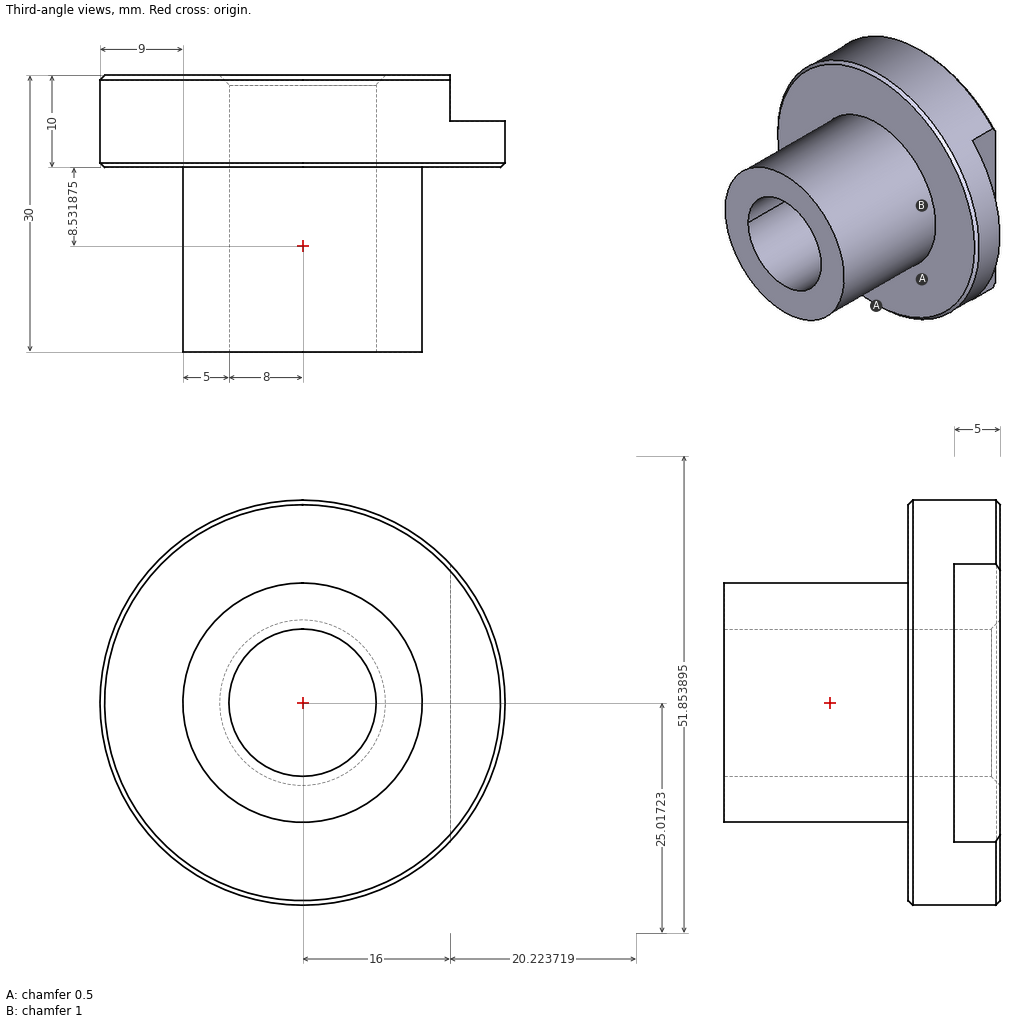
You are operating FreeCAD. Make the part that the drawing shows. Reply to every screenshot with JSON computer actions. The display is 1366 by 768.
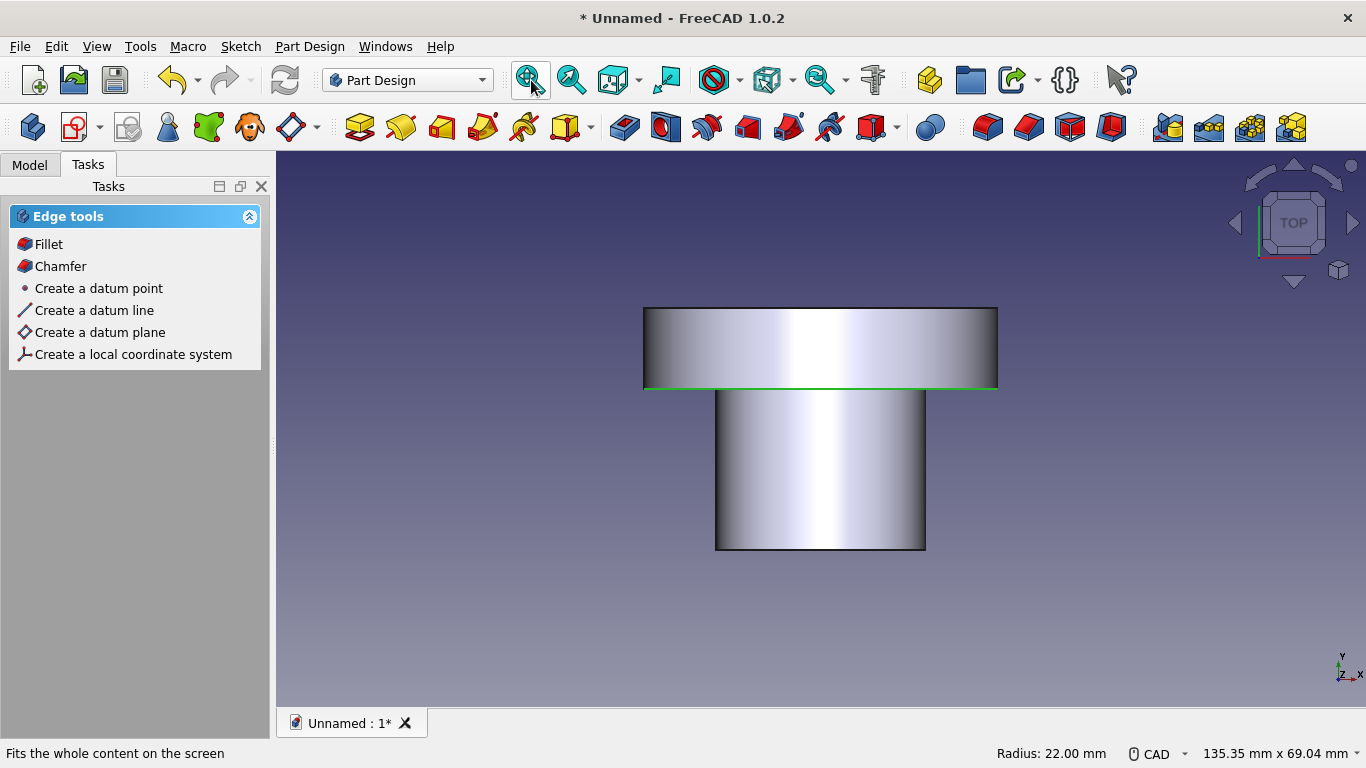
{"action": "left_click", "coordinate": [964, 307], "text": "ctrl"}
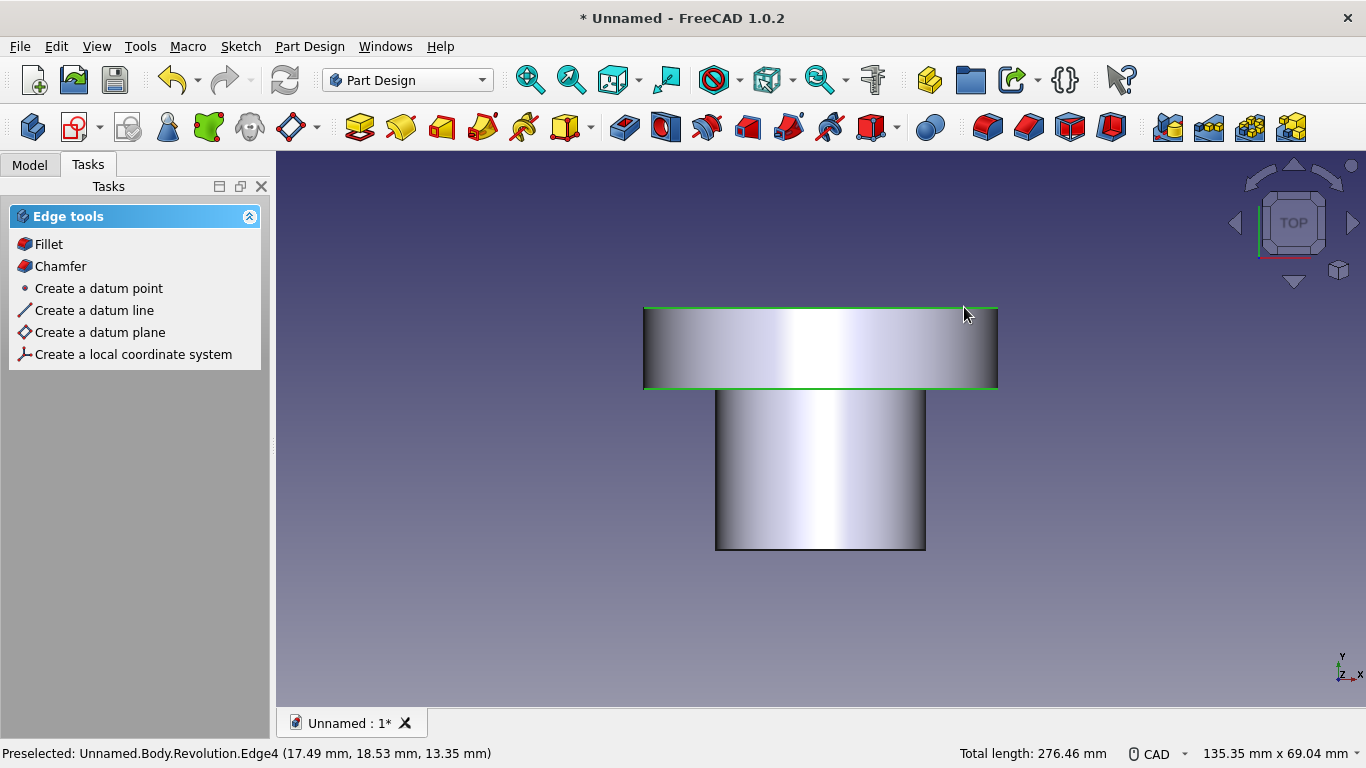
{"action": "left_click", "coordinate": [1029, 128]}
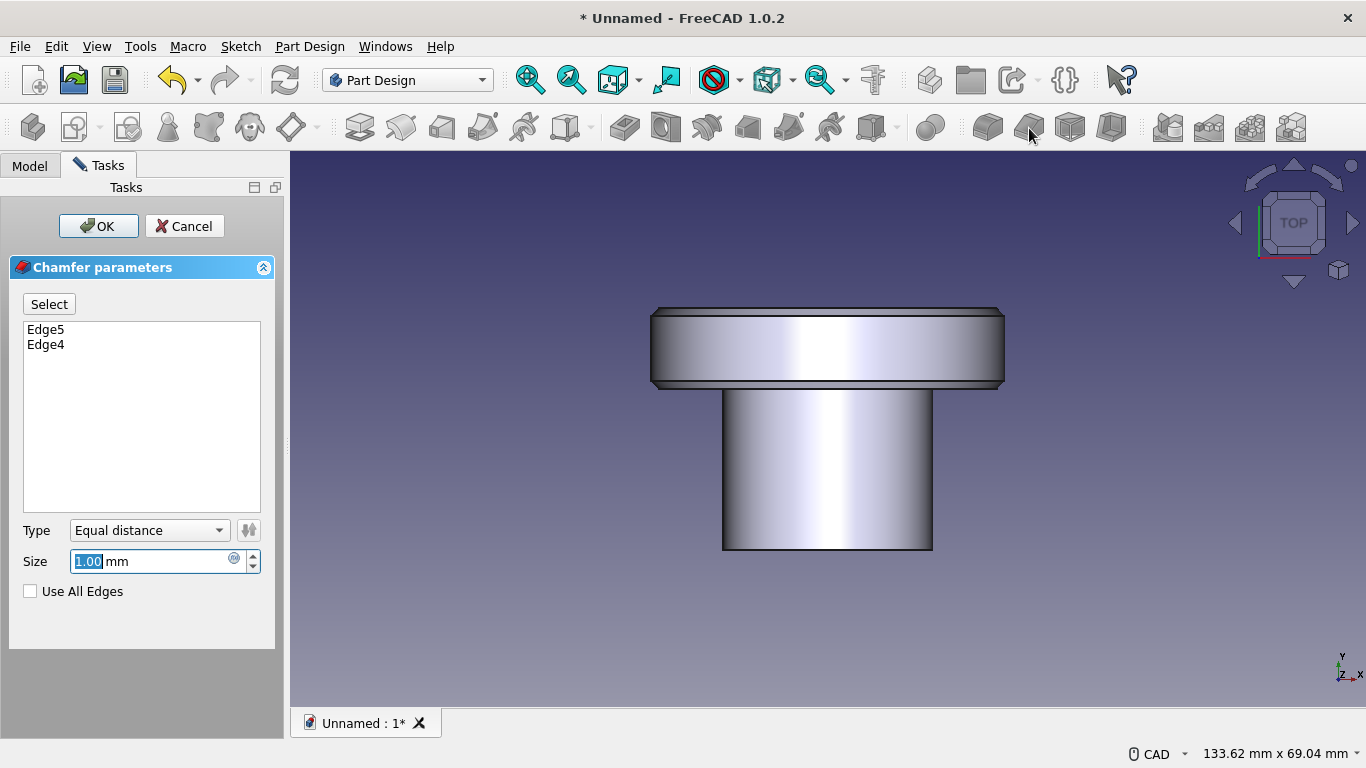
{"action": "type", "text": "0.5"}
{"action": "key", "text": "Tab"}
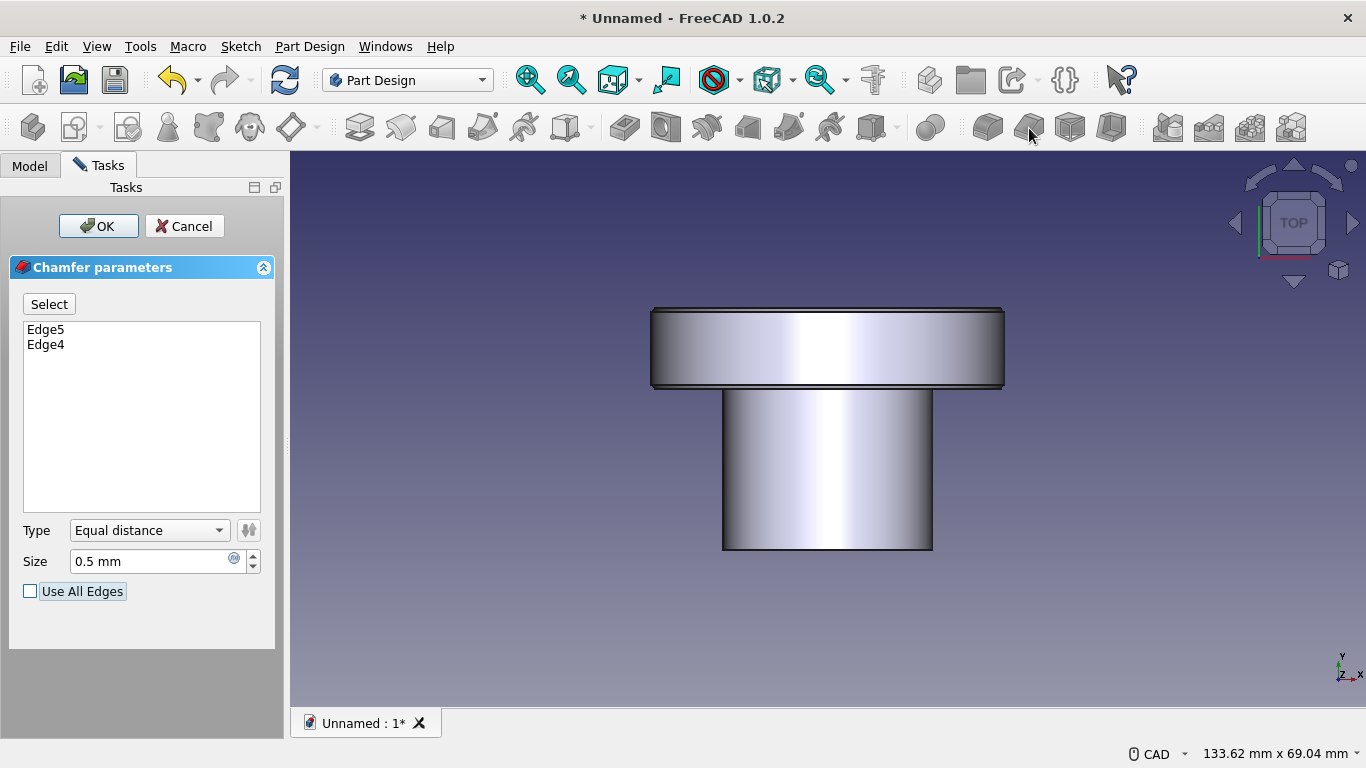
{"action": "left_click", "coordinate": [99, 226]}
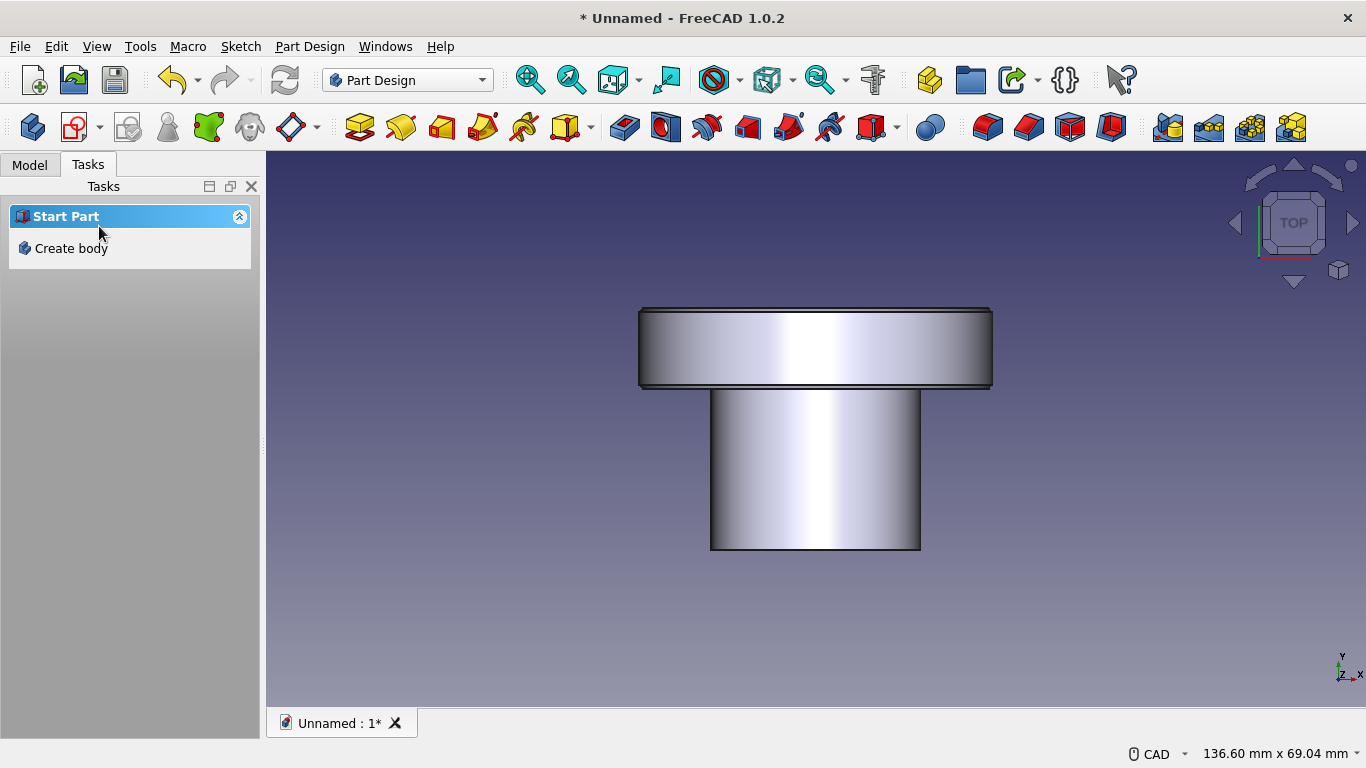
{"action": "left_click", "coordinate": [531, 80]}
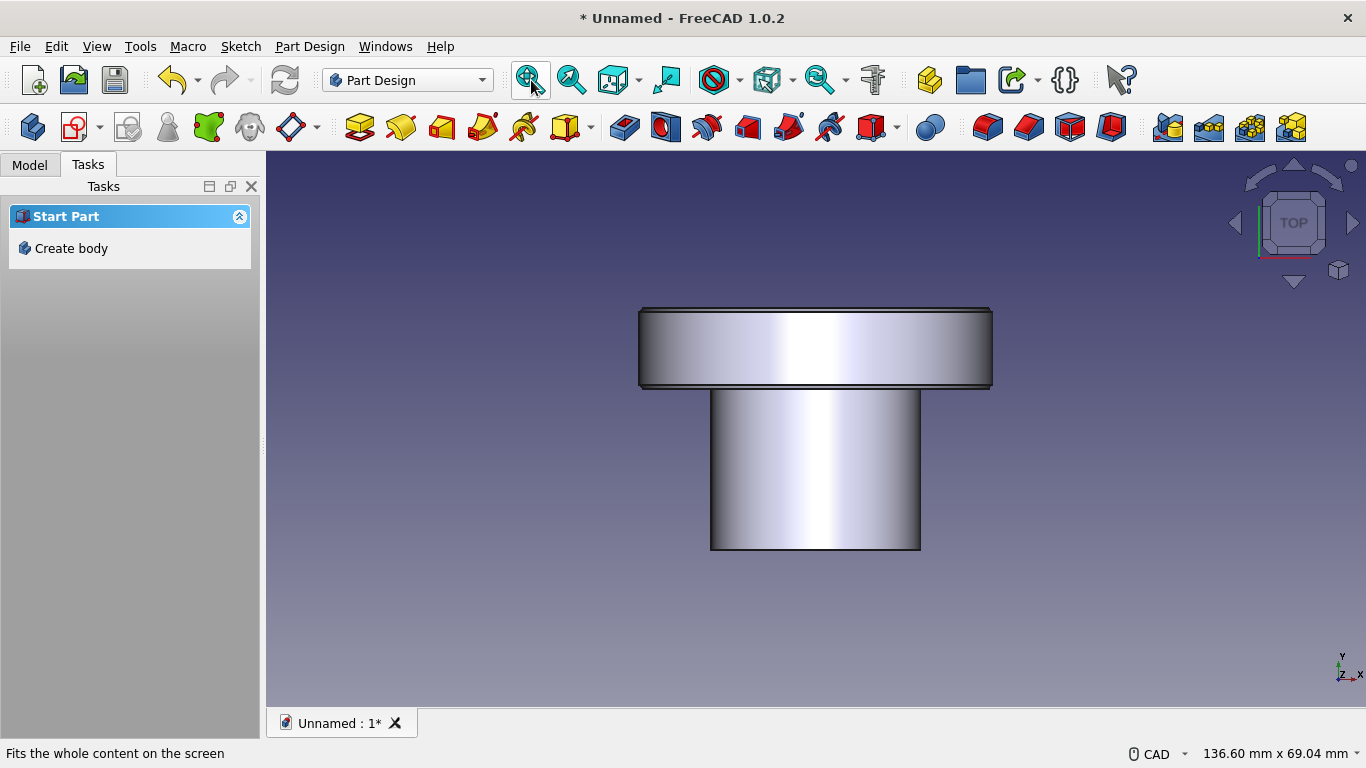
{"action": "key", "text": "0"}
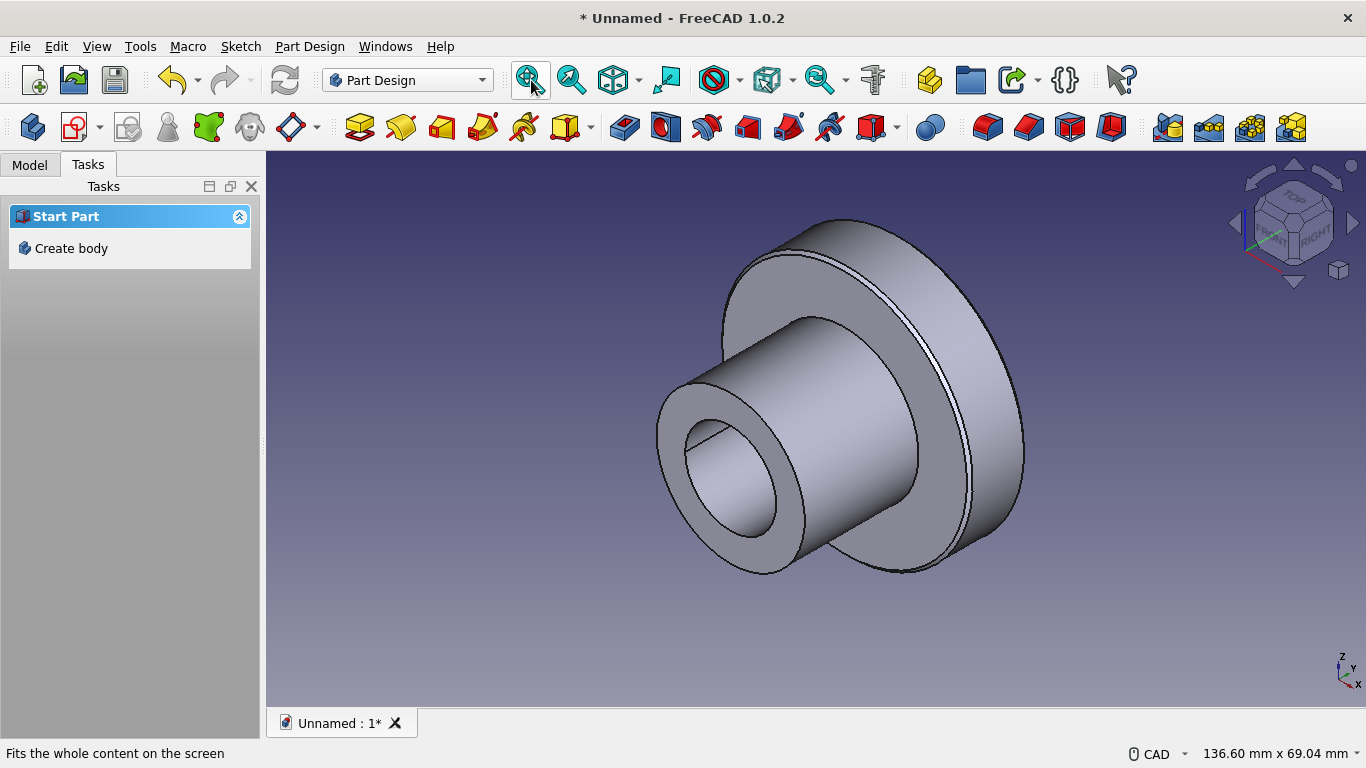
{"action": "key", "text": "2"}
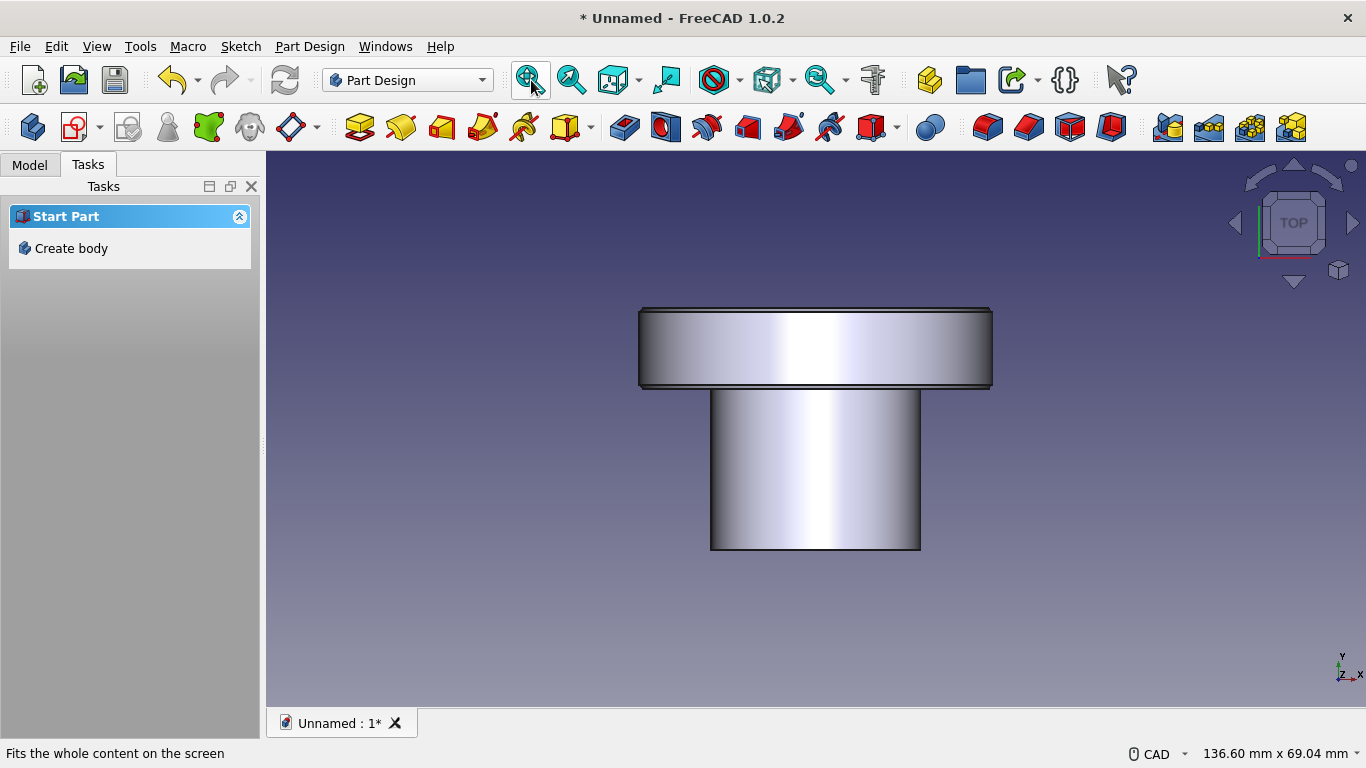
{"action": "left_click", "coordinate": [531, 80]}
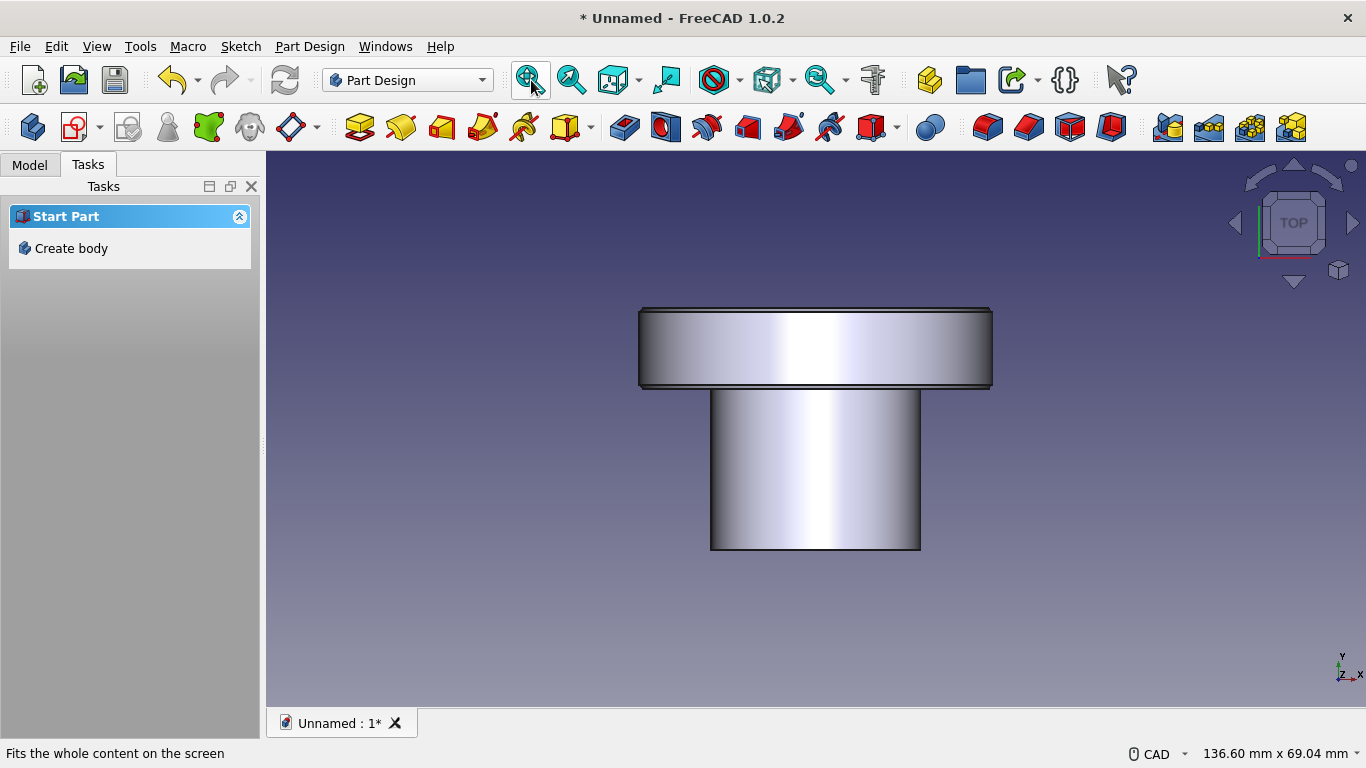
{"action": "key", "text": "1"}